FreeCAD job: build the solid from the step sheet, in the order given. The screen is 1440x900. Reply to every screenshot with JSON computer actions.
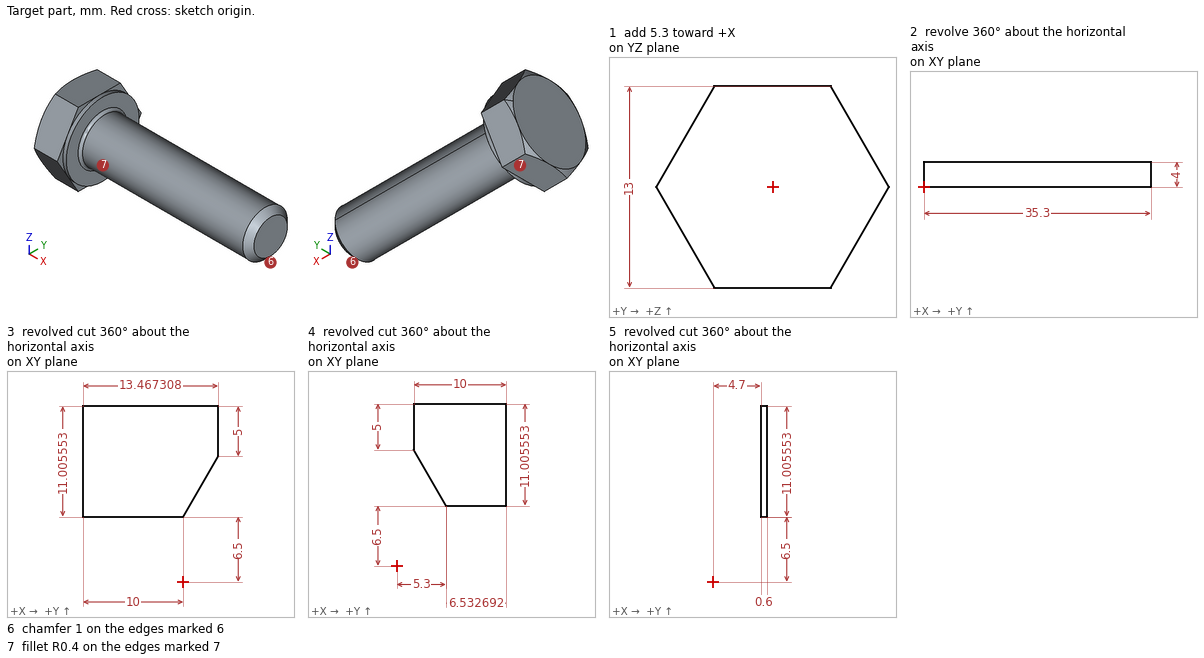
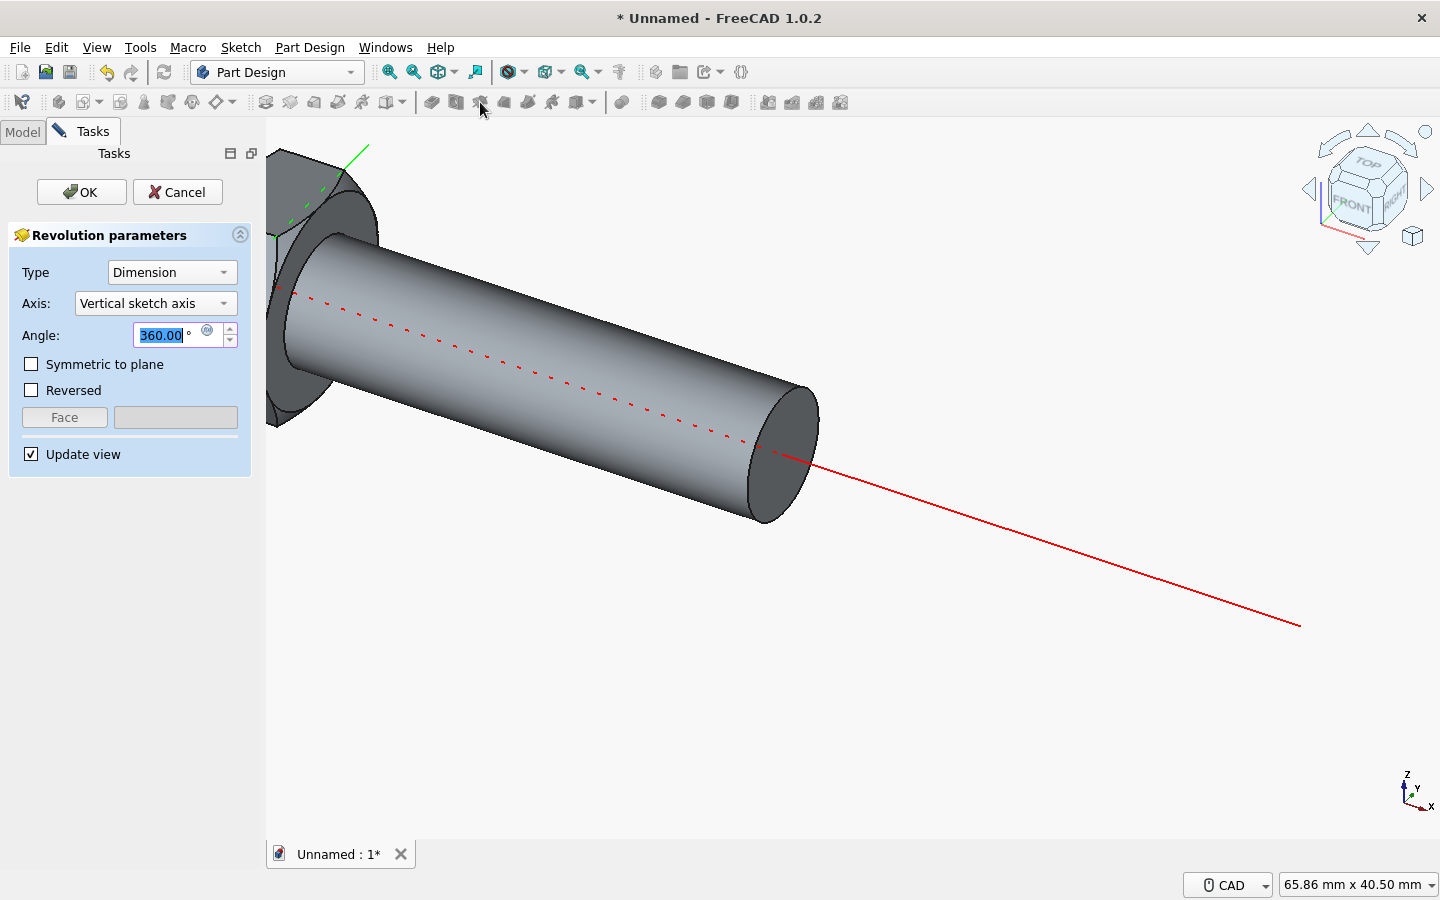
{"action": "left_click", "coordinate": [156, 304]}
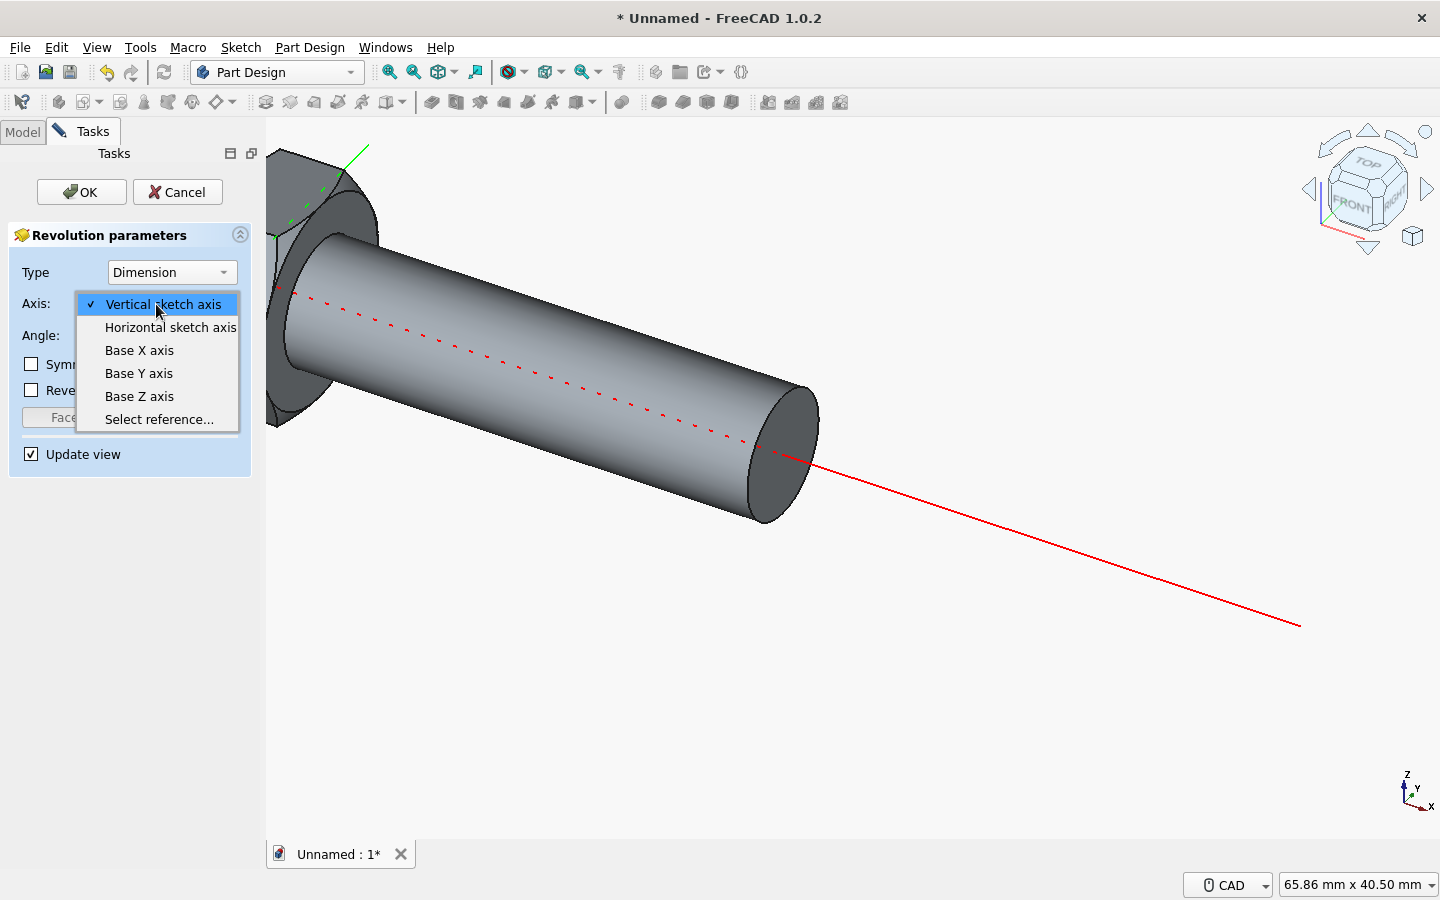
{"action": "left_click", "coordinate": [156, 328]}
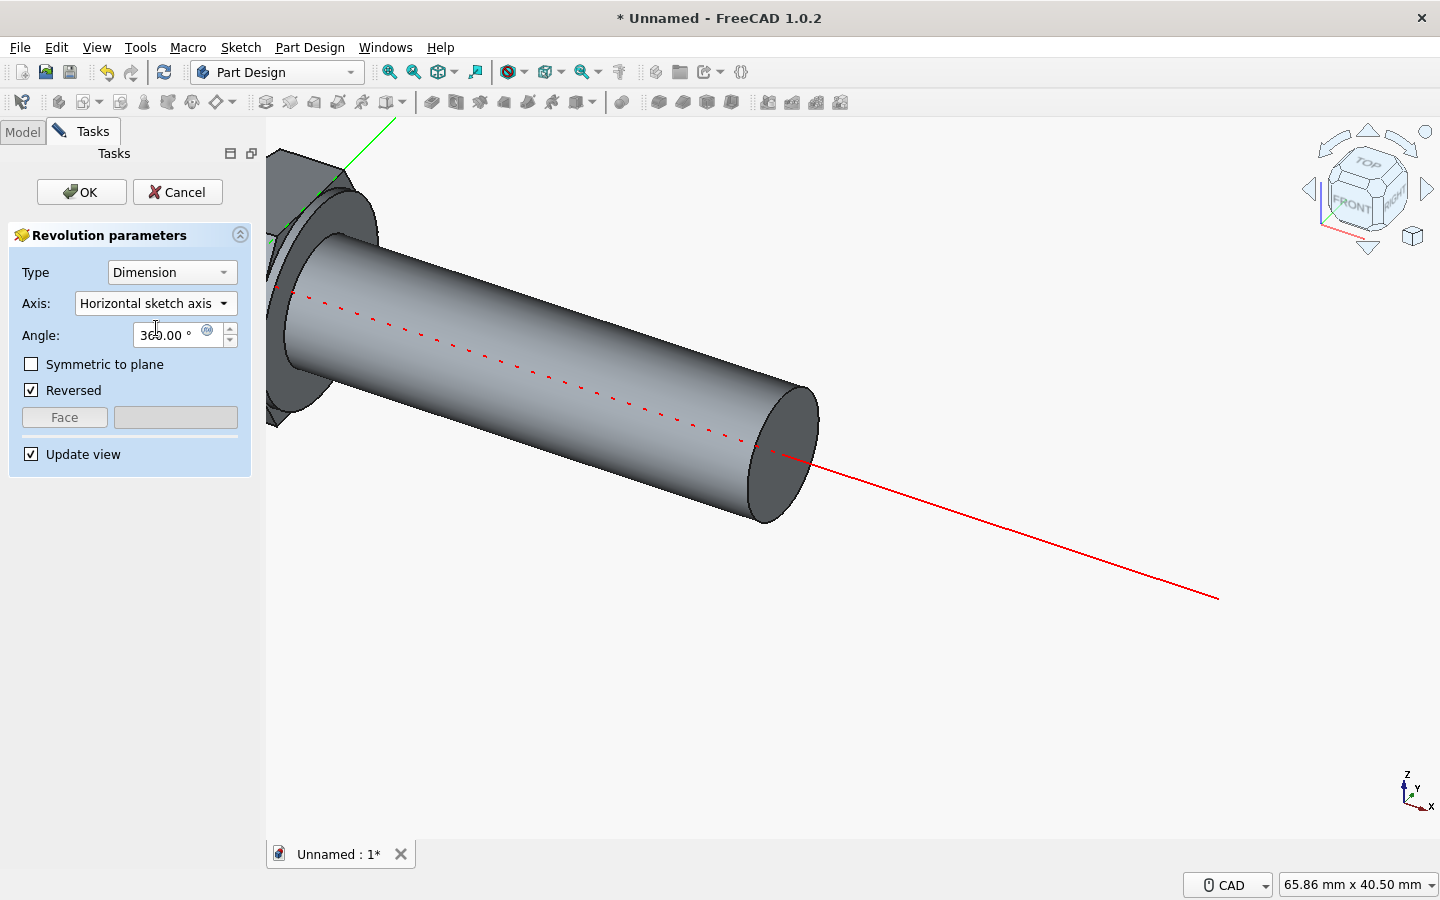
{"action": "left_click", "coordinate": [82, 192]}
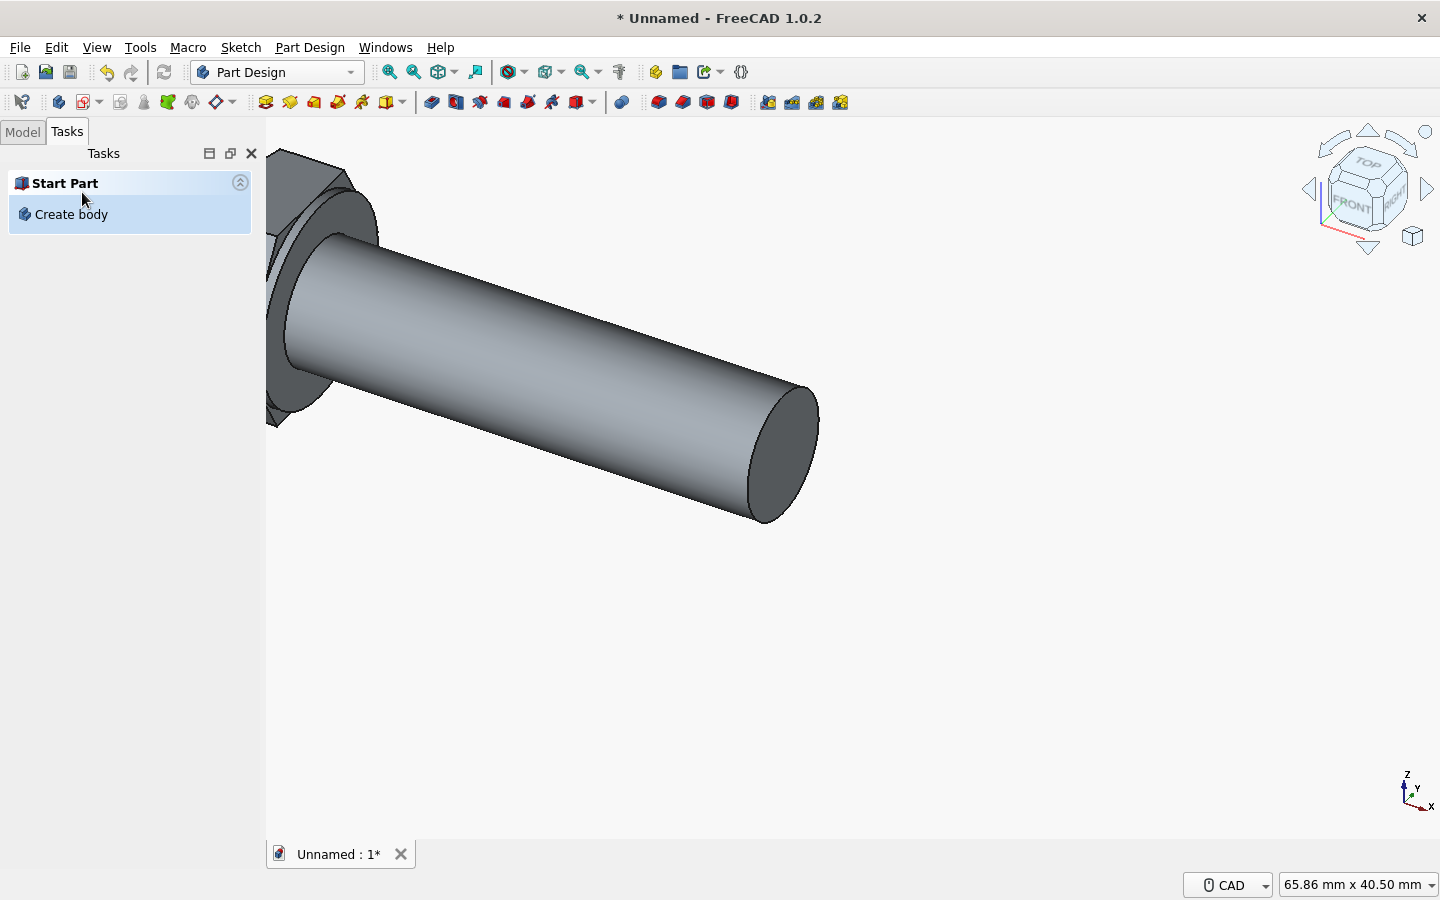
{"action": "key", "text": "v f"}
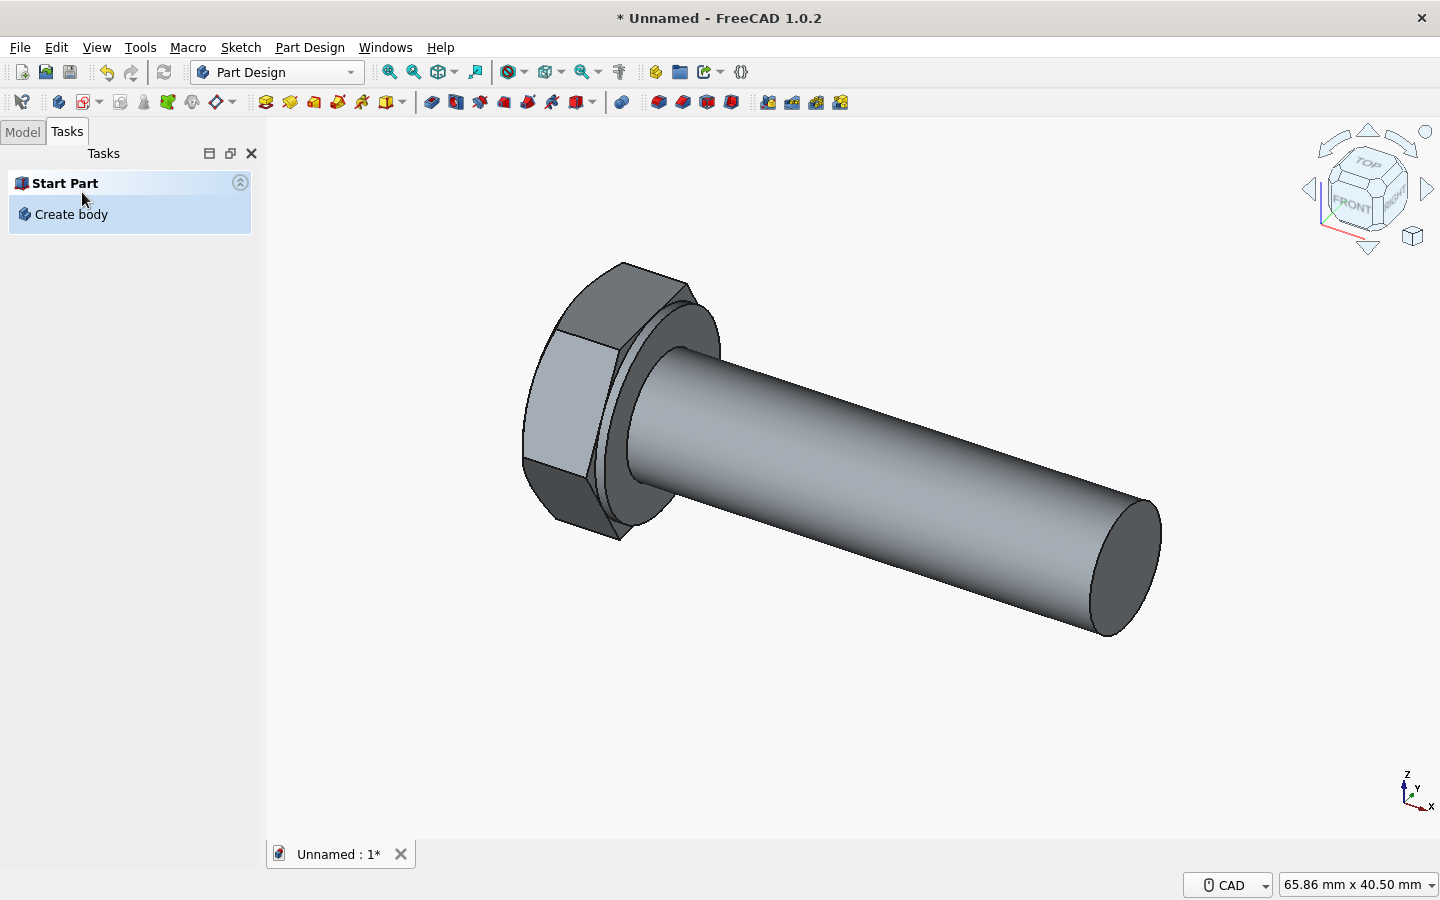
{"action": "left_click", "coordinate": [1090, 603]}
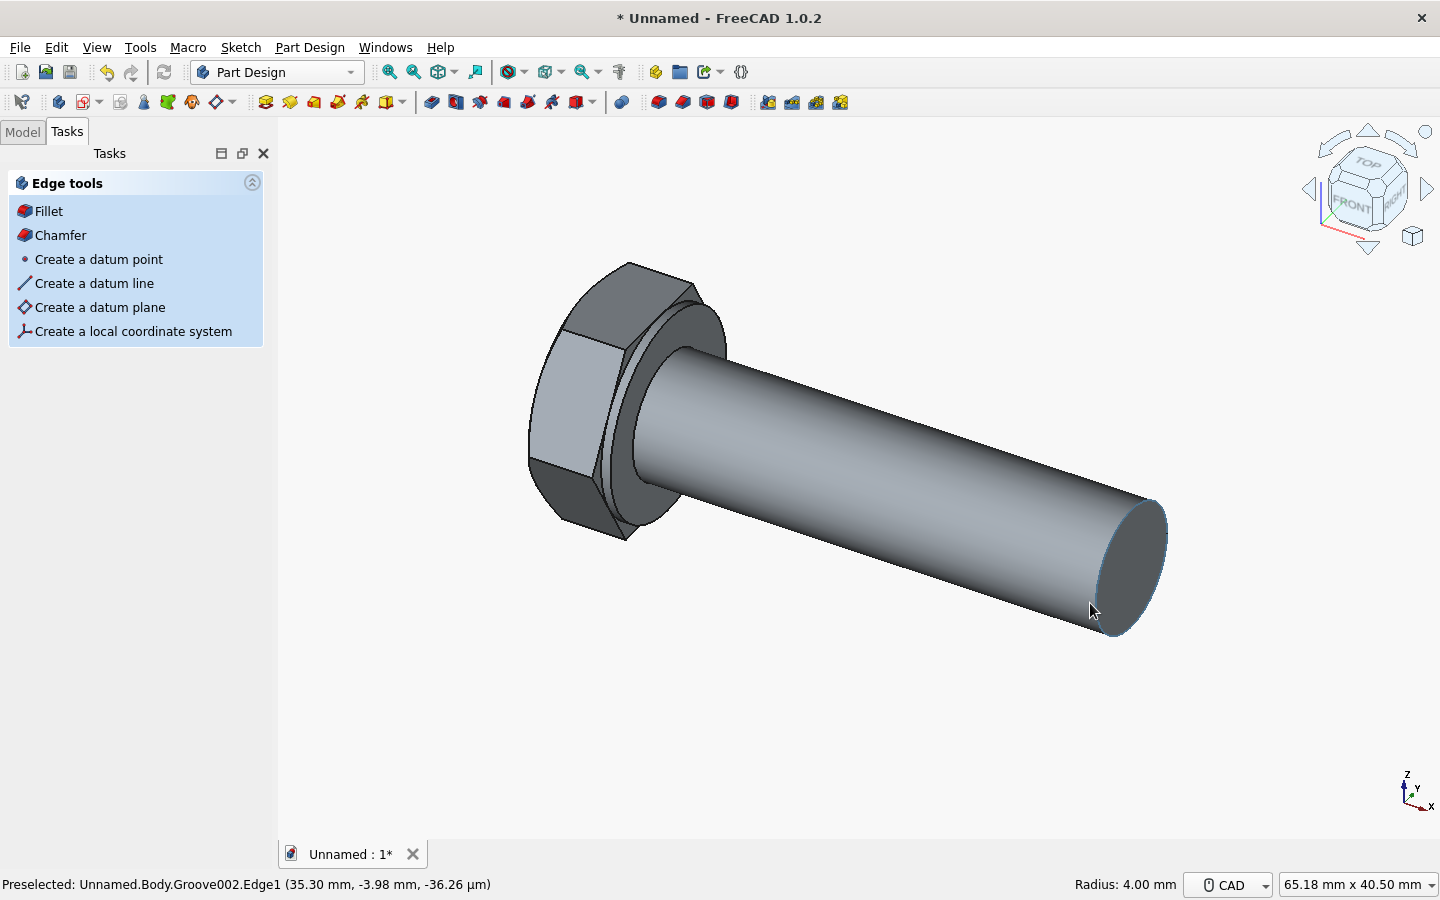
{"action": "left_click", "coordinate": [684, 102]}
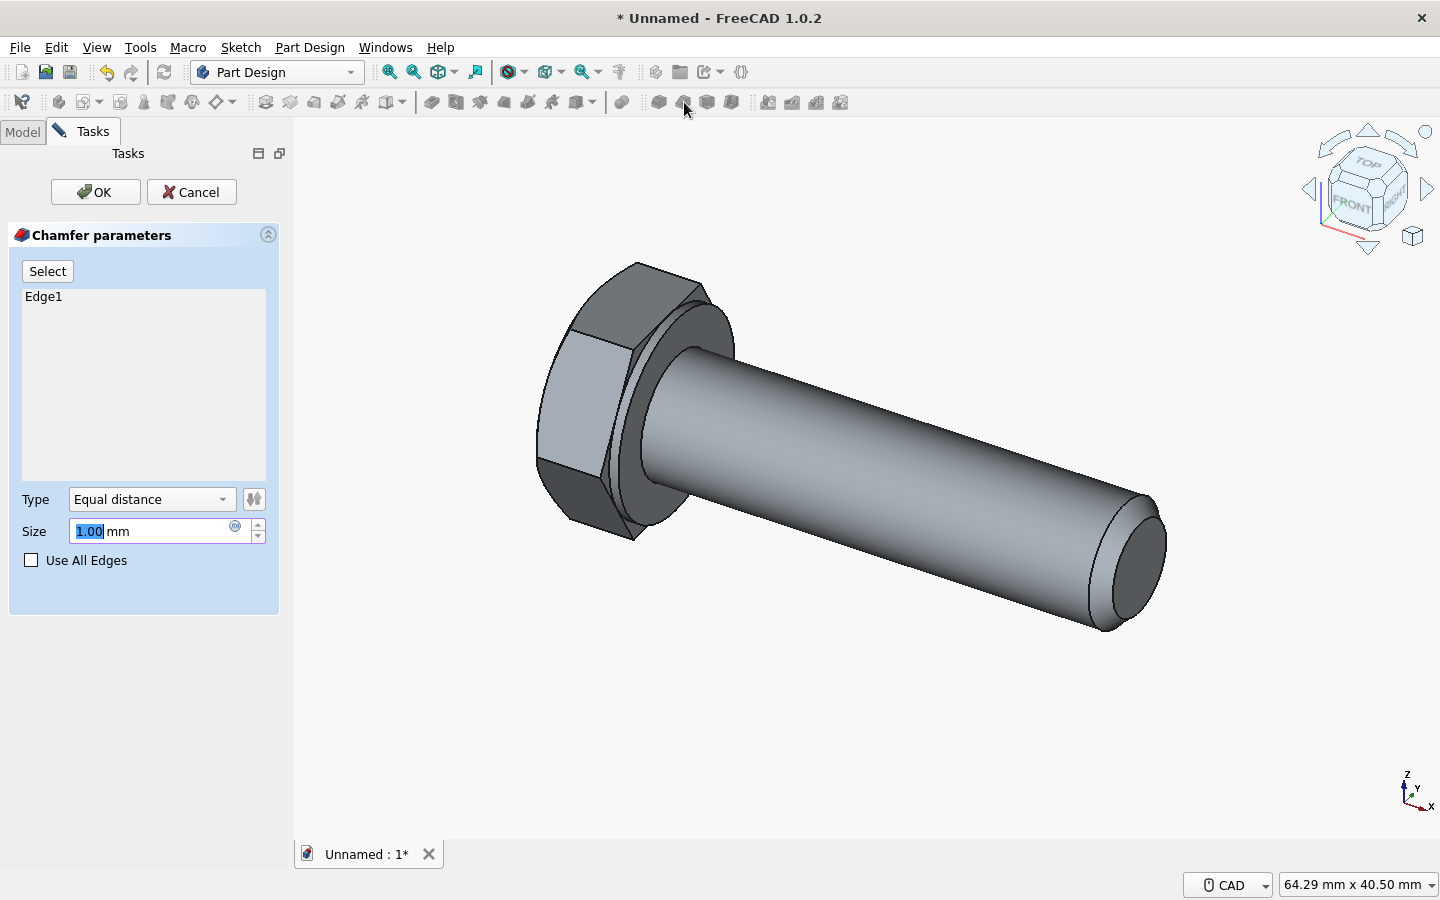
{"action": "type", "text": "1"}
{"action": "key", "text": "Tab"}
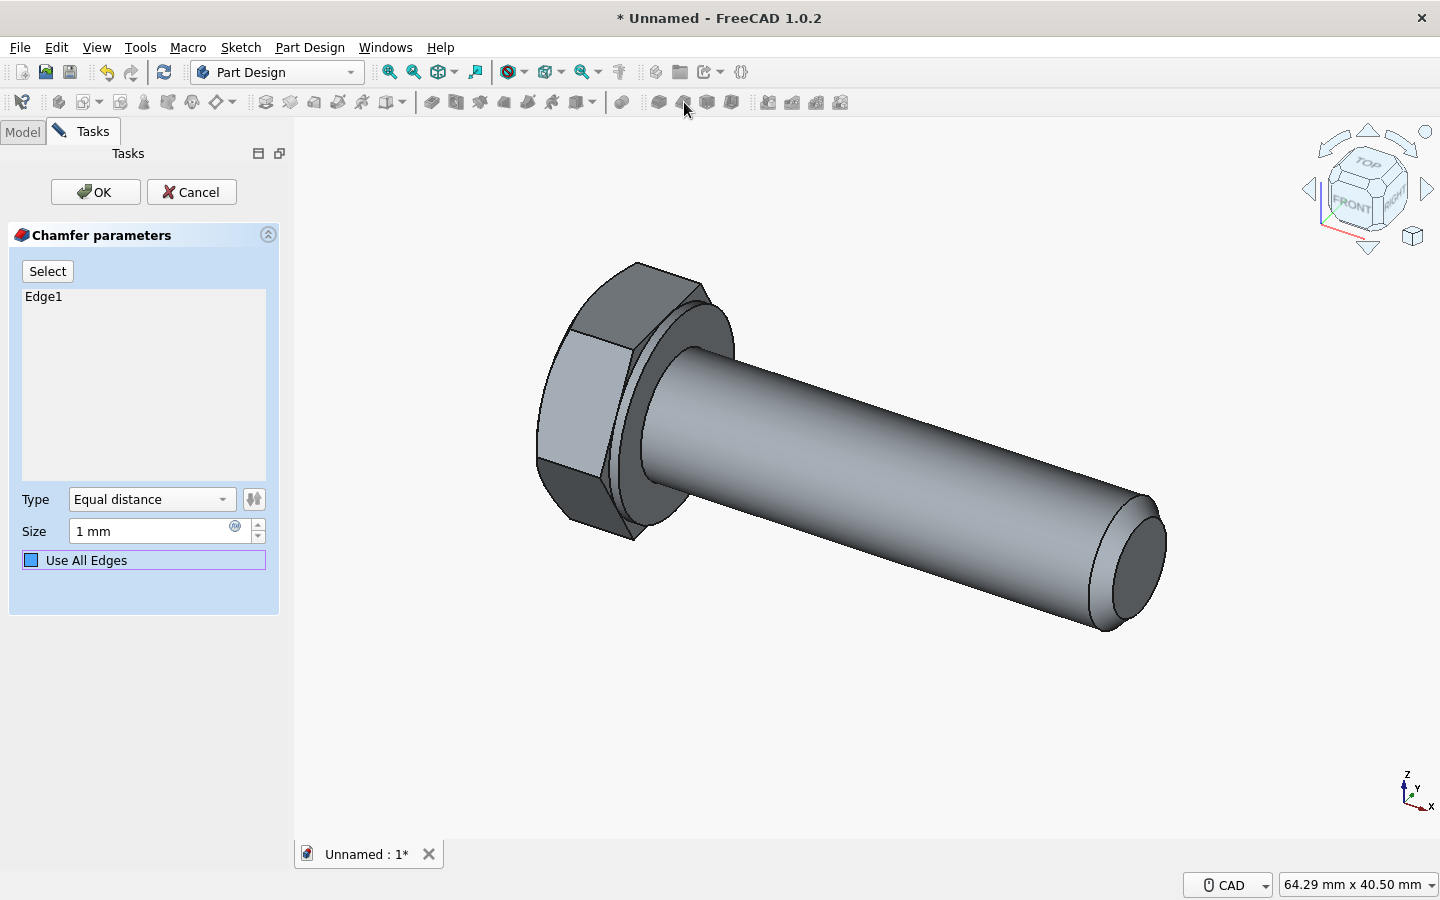
{"action": "left_click", "coordinate": [96, 192]}